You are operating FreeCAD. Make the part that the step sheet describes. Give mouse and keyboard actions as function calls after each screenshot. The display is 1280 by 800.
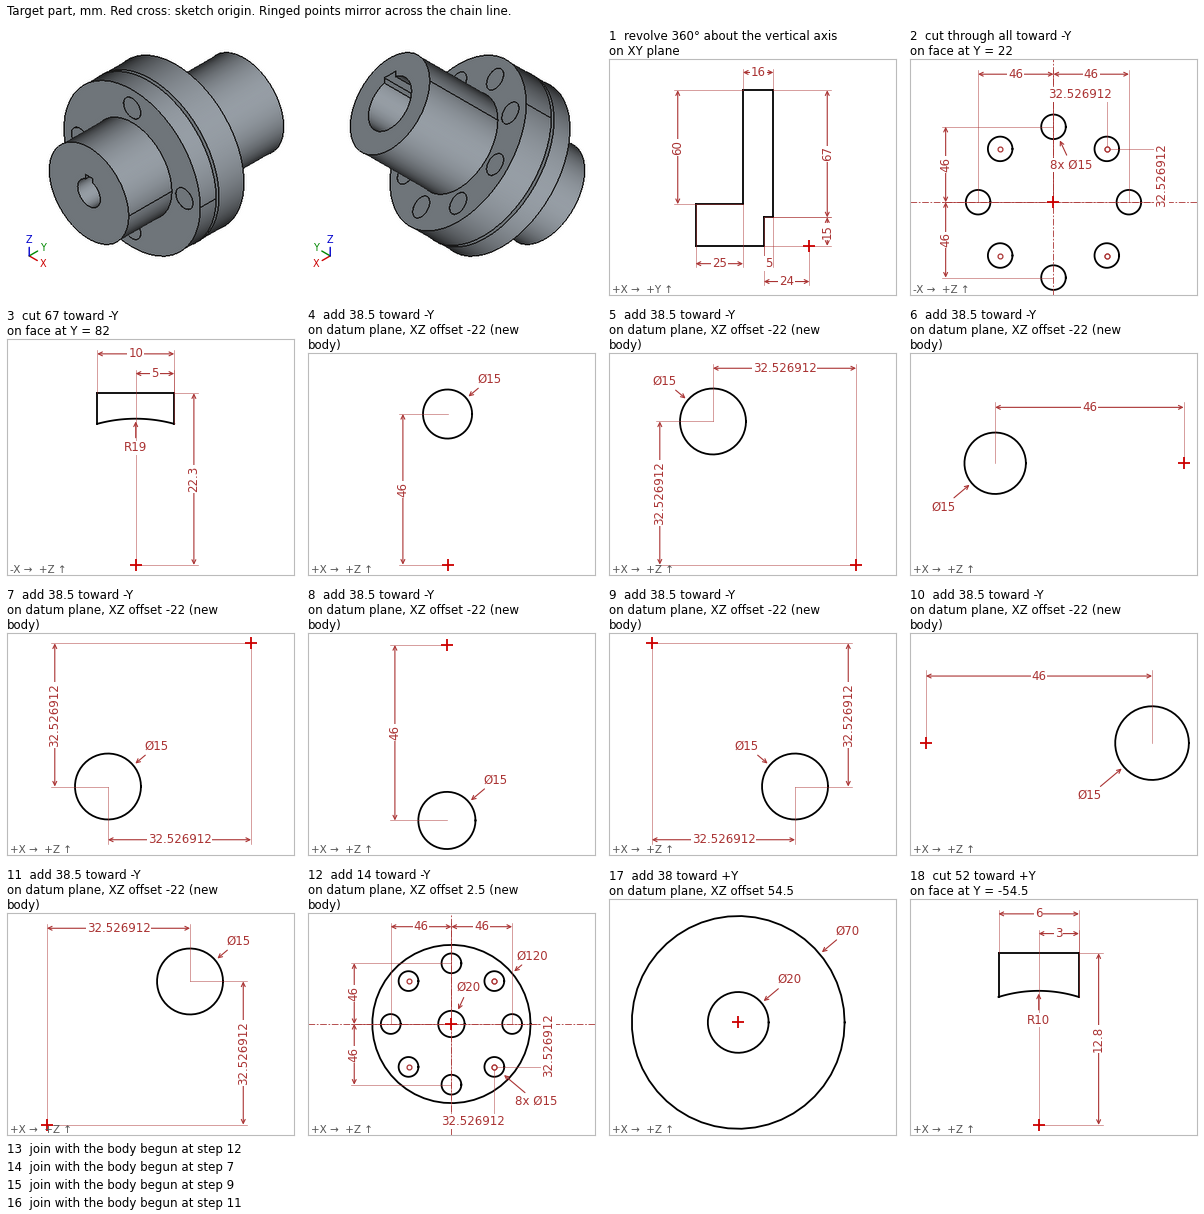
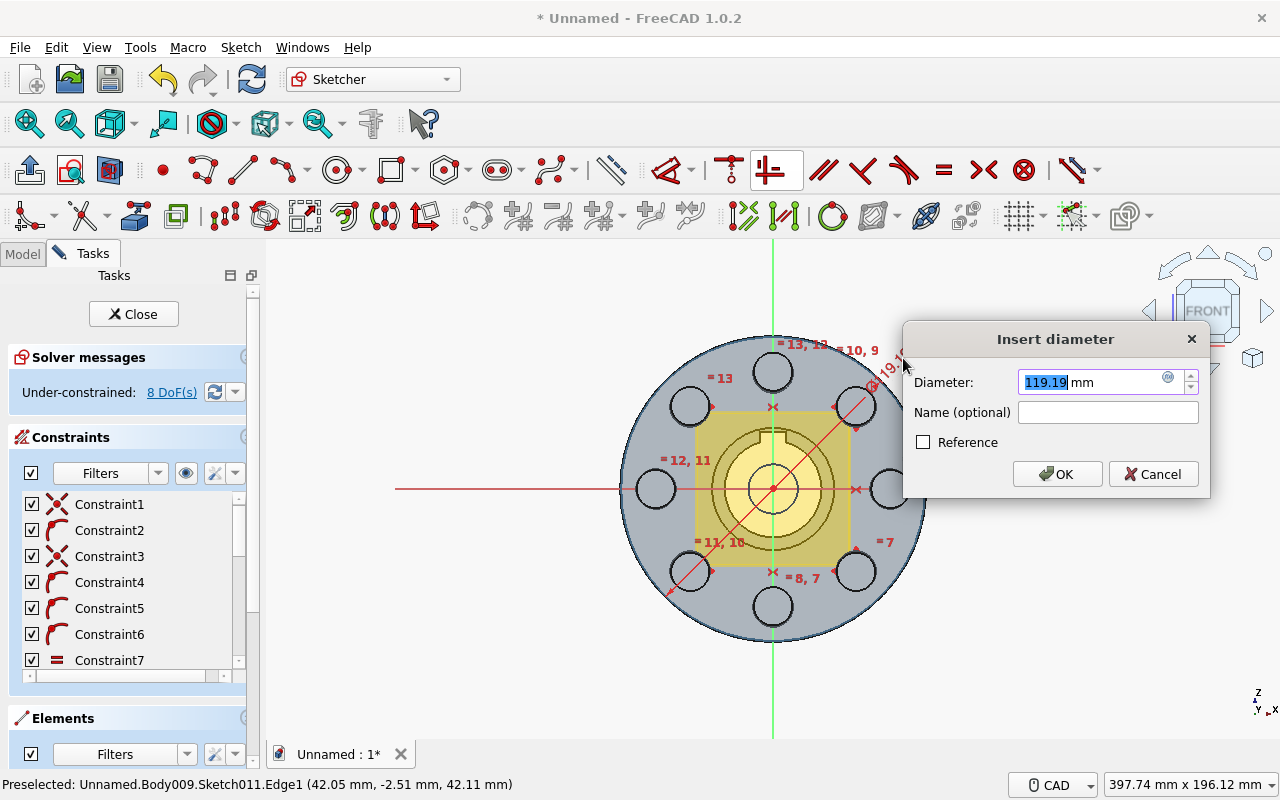
text(120)
key(Return)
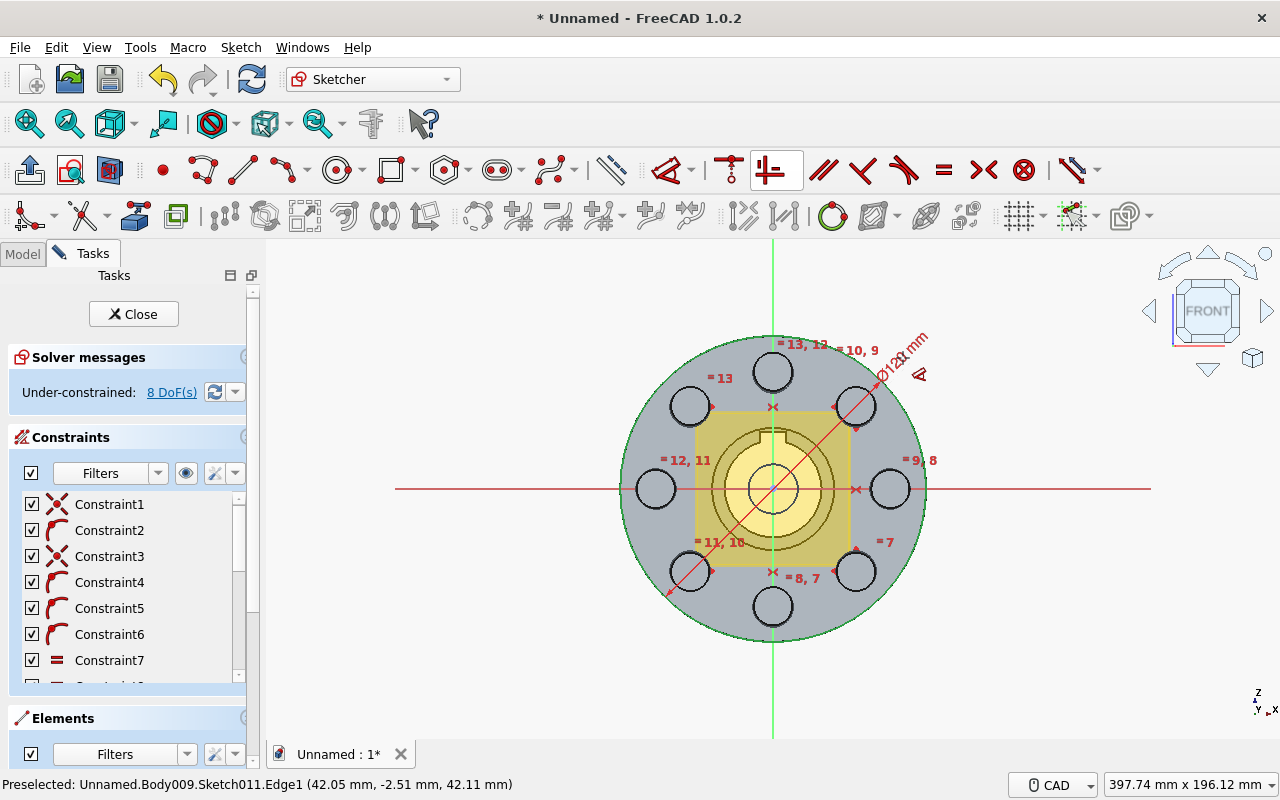
click(870, 557)
click(892, 534)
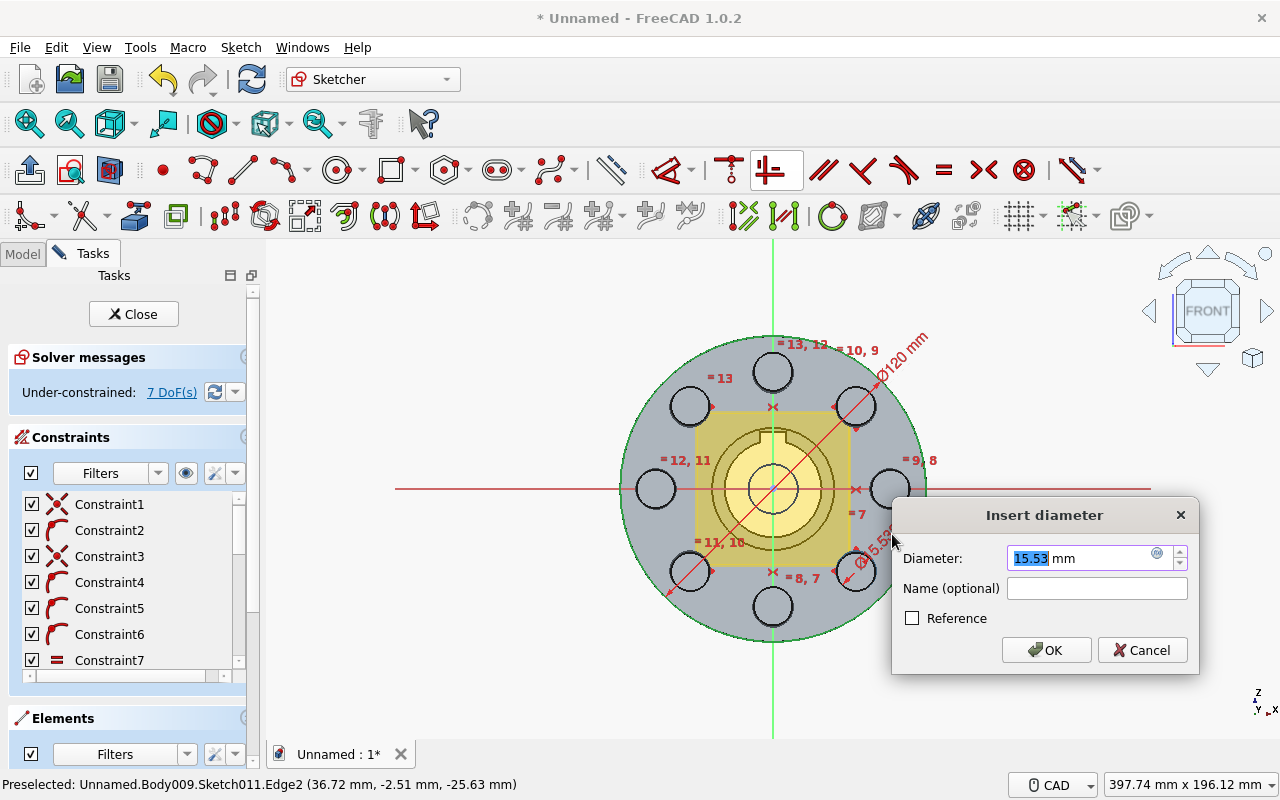
text(15)
key(Return)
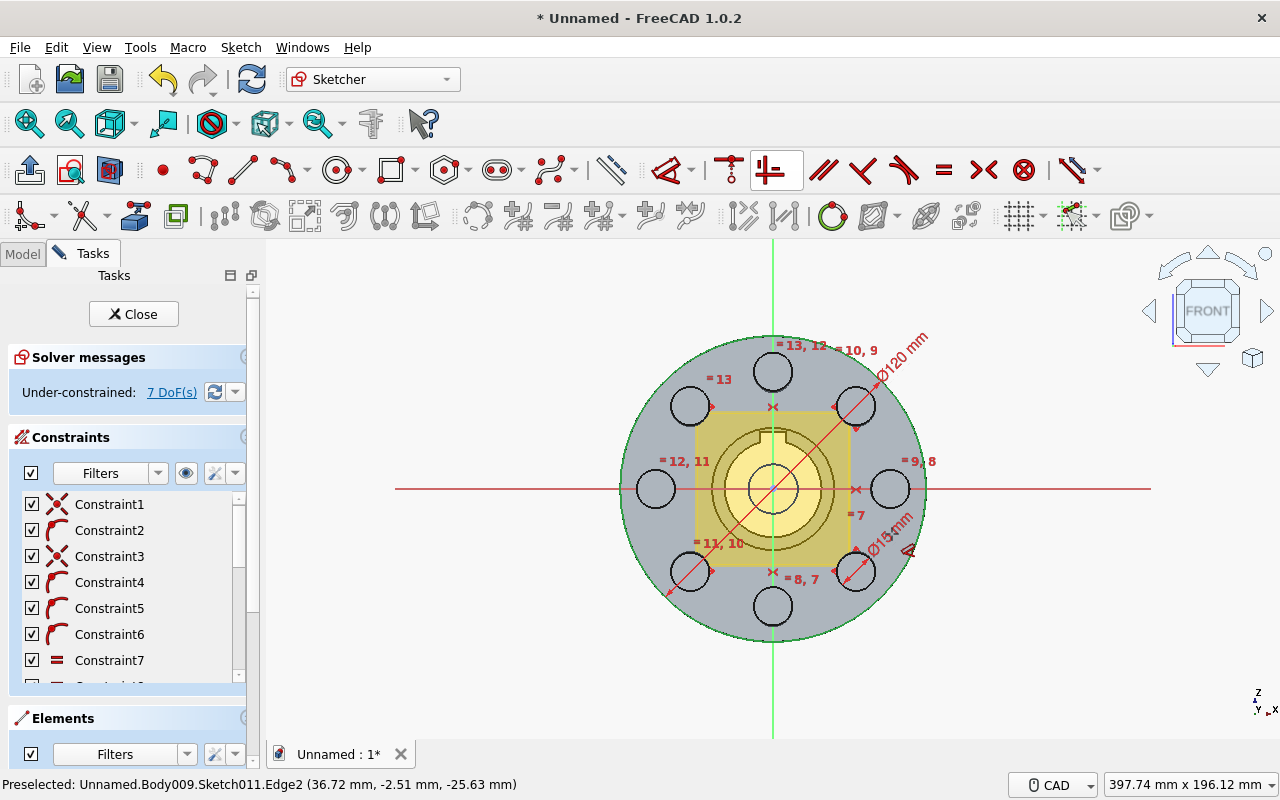
click(791, 472)
click(814, 450)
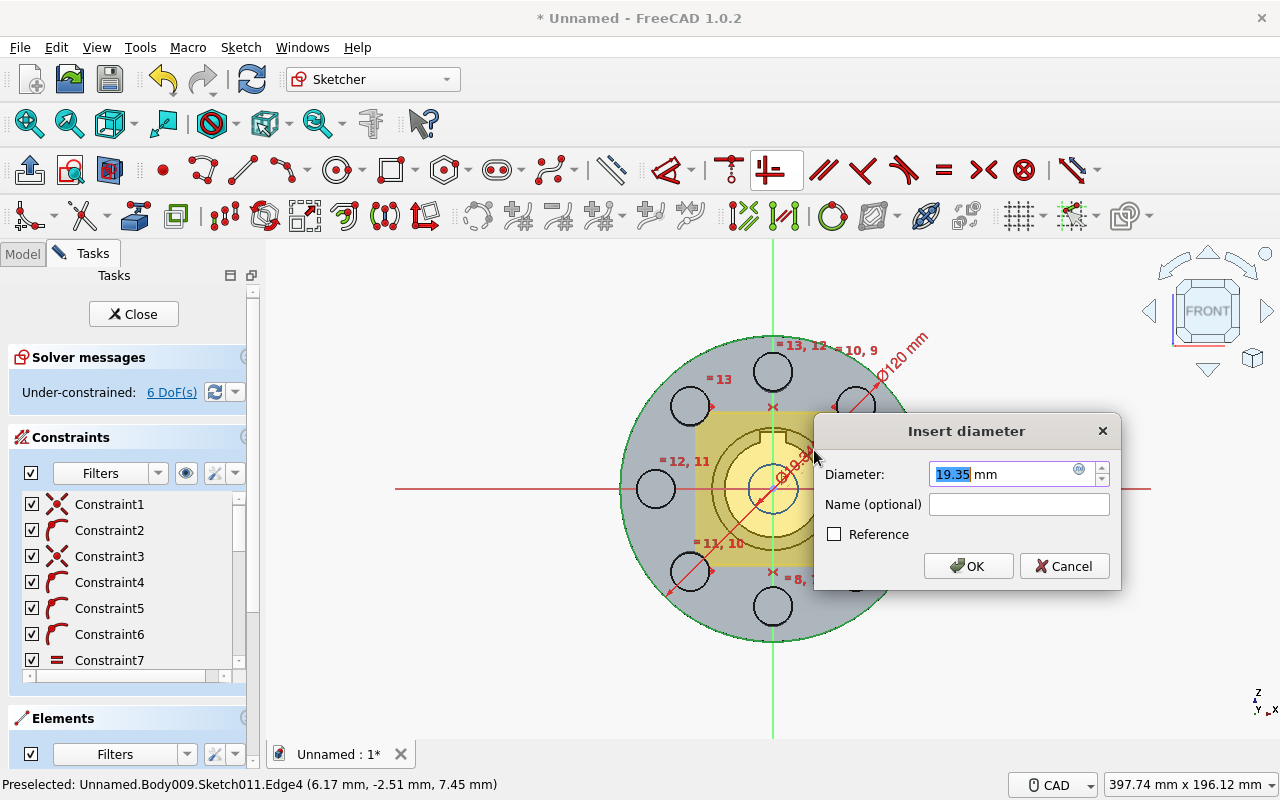
text(20)
key(Return)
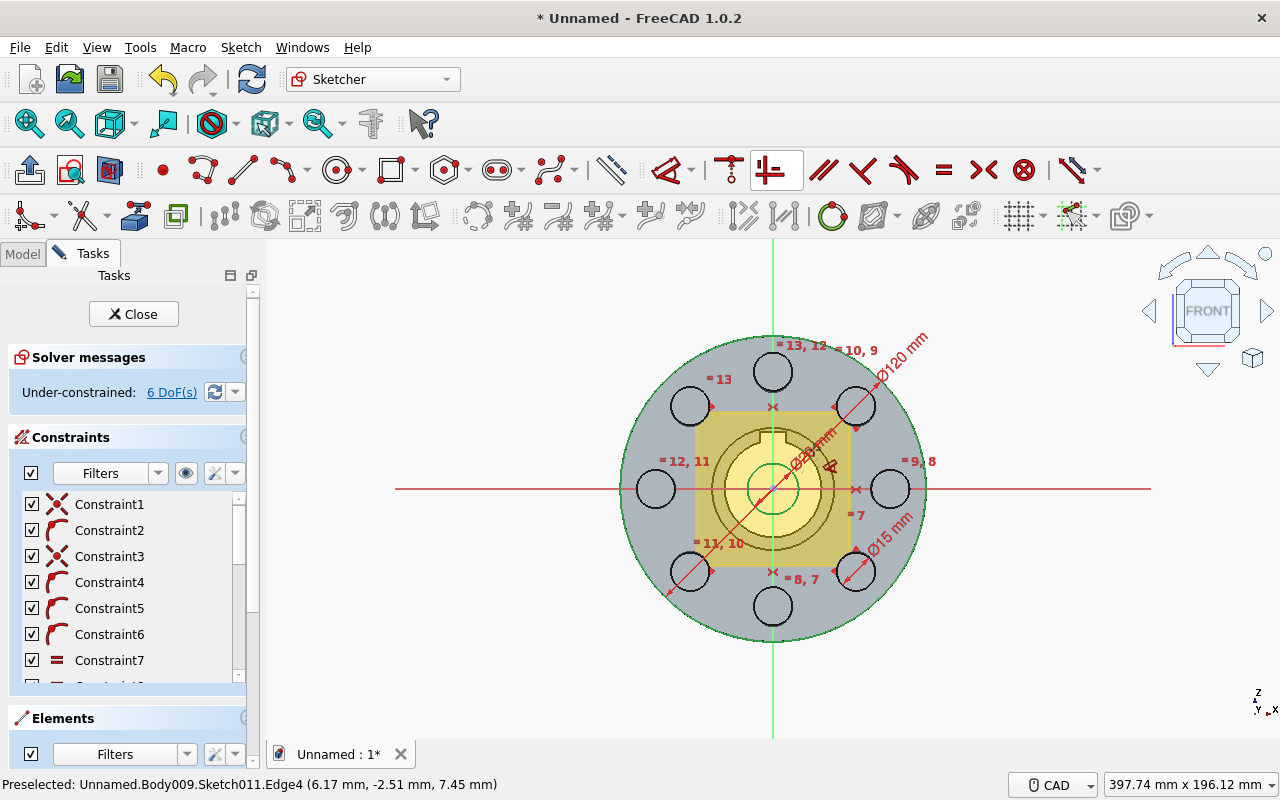
click(773, 607)
click(807, 548)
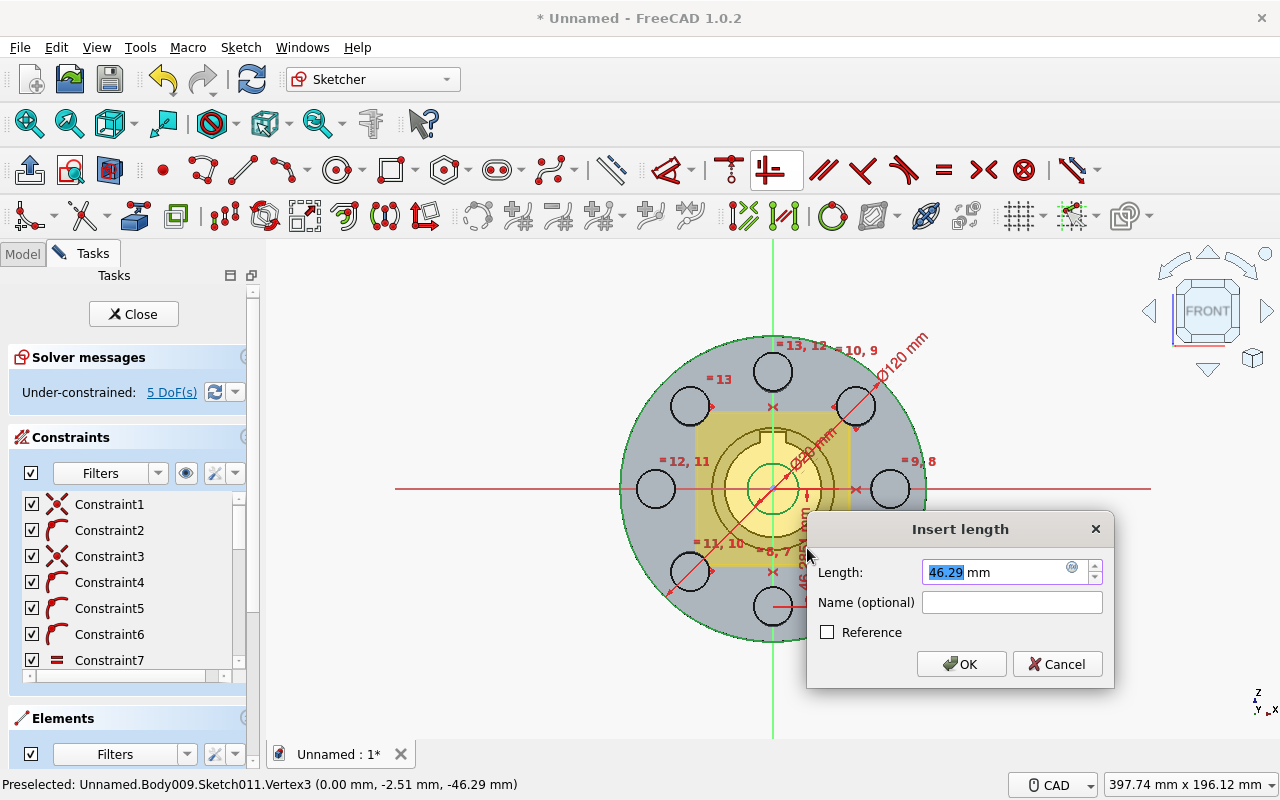
text(46)
key(Return)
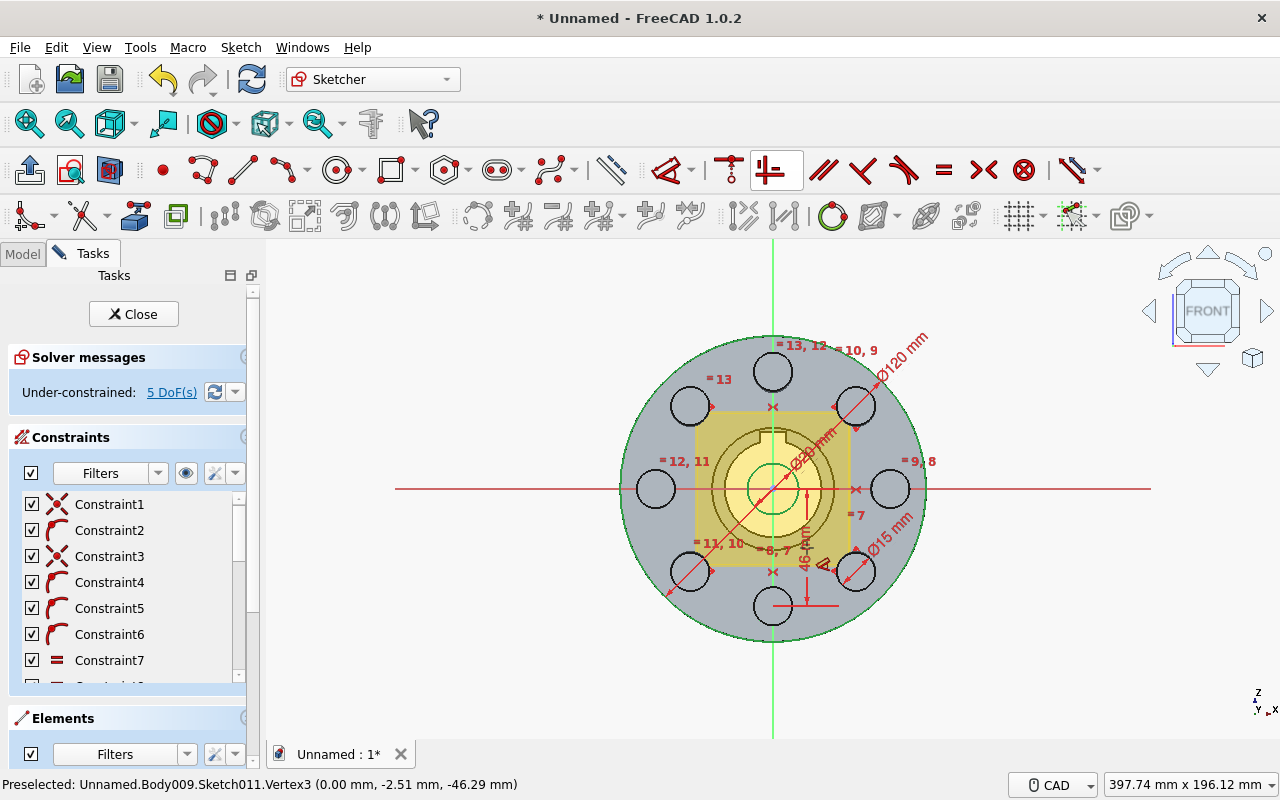
click(890, 489)
click(805, 523)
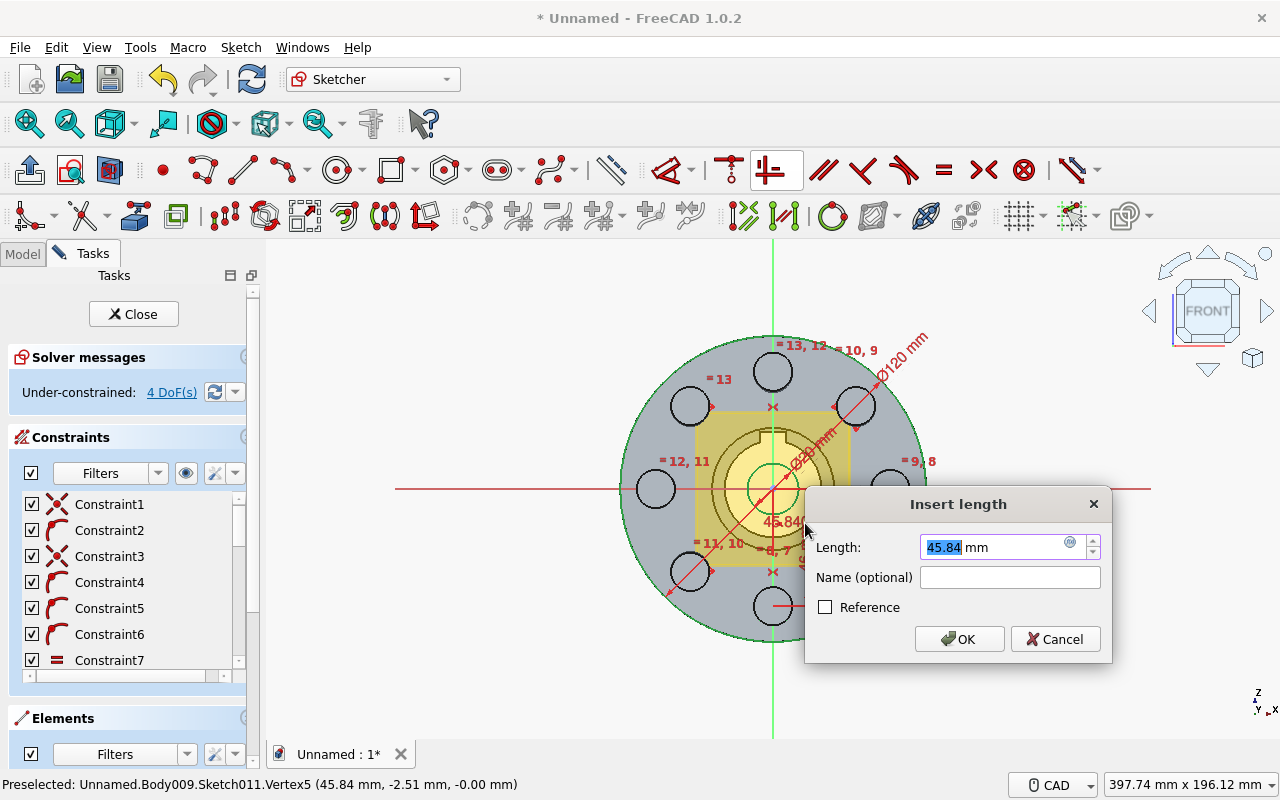
text(46)
key(Return)